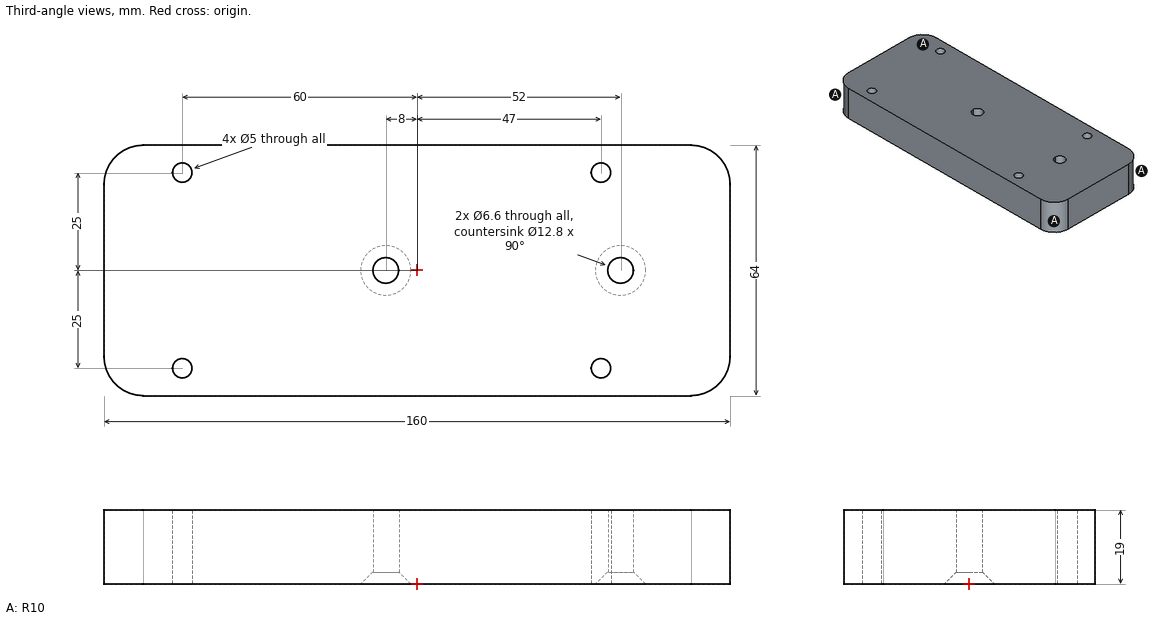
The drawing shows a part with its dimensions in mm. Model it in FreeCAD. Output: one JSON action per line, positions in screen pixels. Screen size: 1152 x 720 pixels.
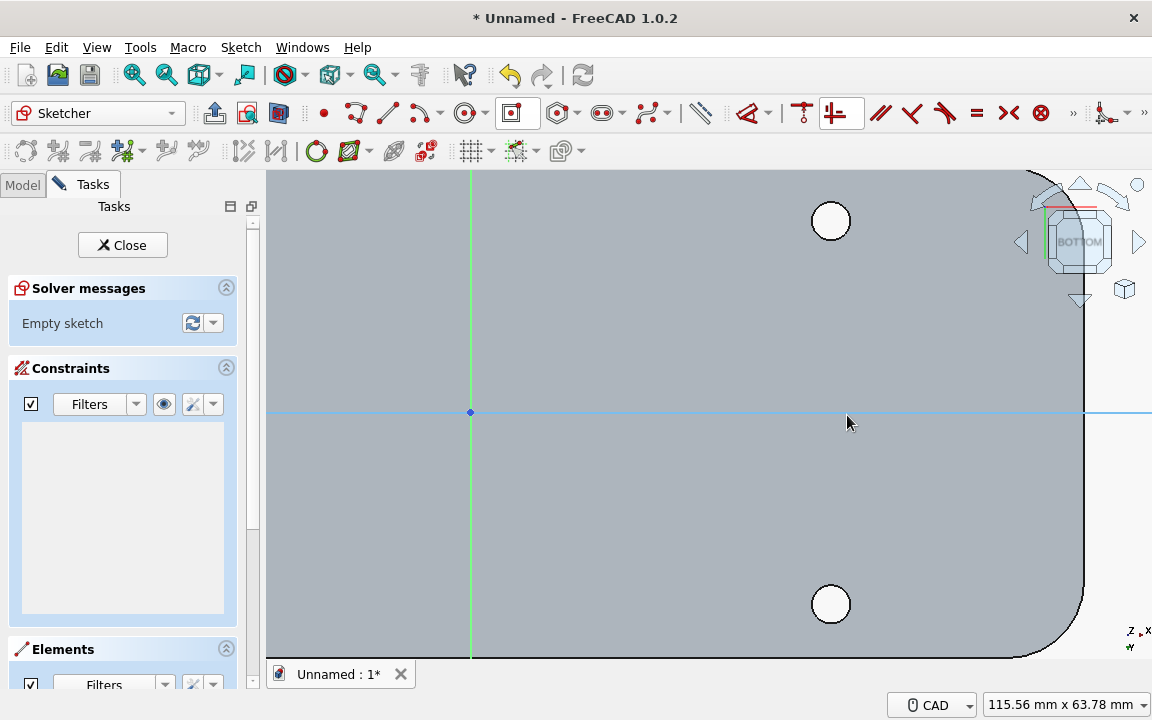
{"action": "left_click", "coordinate": [466, 114]}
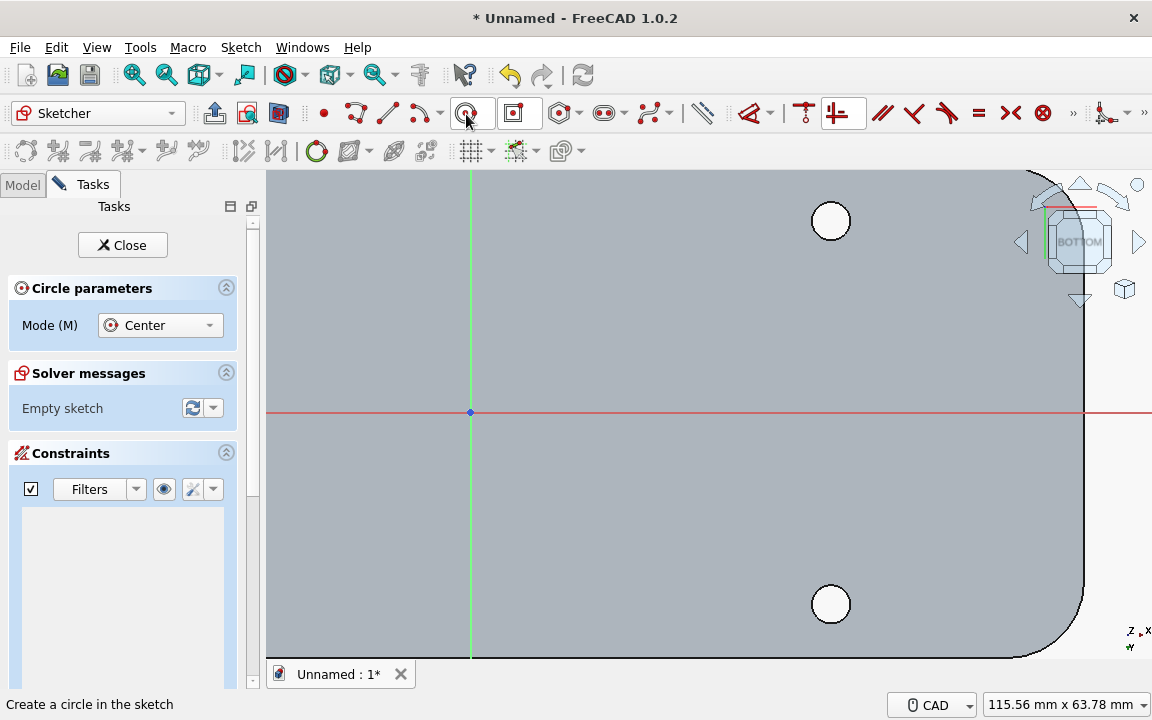
{"action": "left_click", "coordinate": [869, 413]}
{"action": "left_click", "coordinate": [887, 395]}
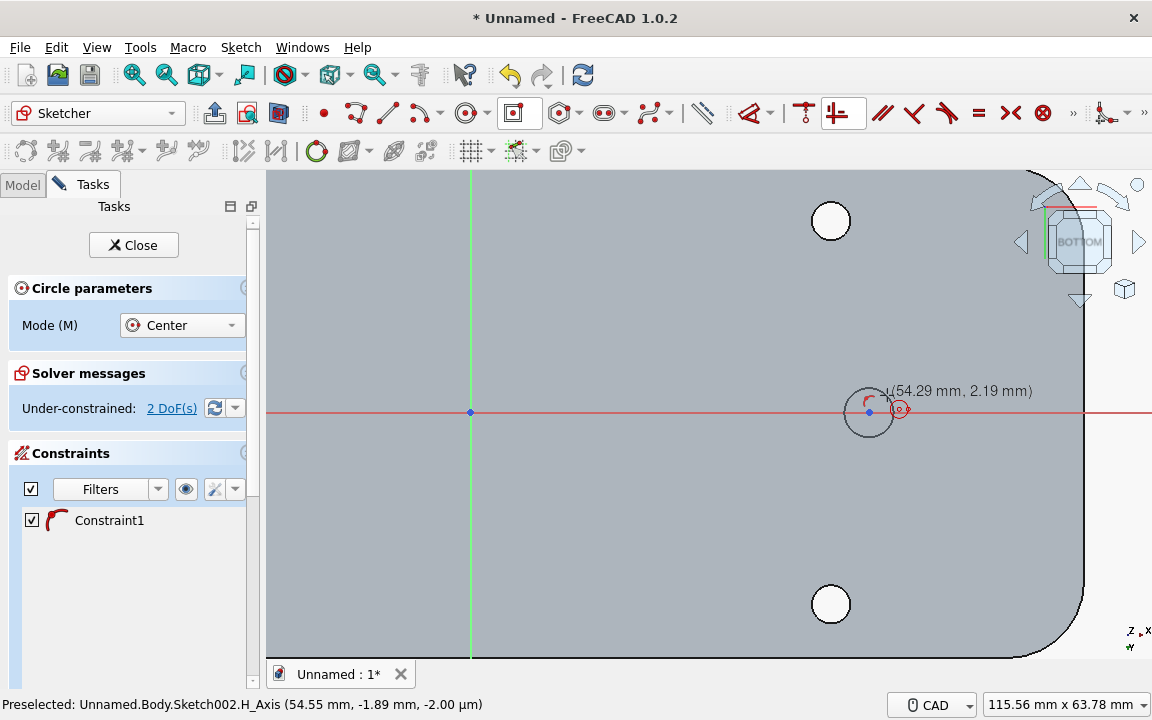
{"action": "left_click", "coordinate": [409, 413]}
{"action": "left_click", "coordinate": [427, 395]}
{"action": "key", "text": "Escape"}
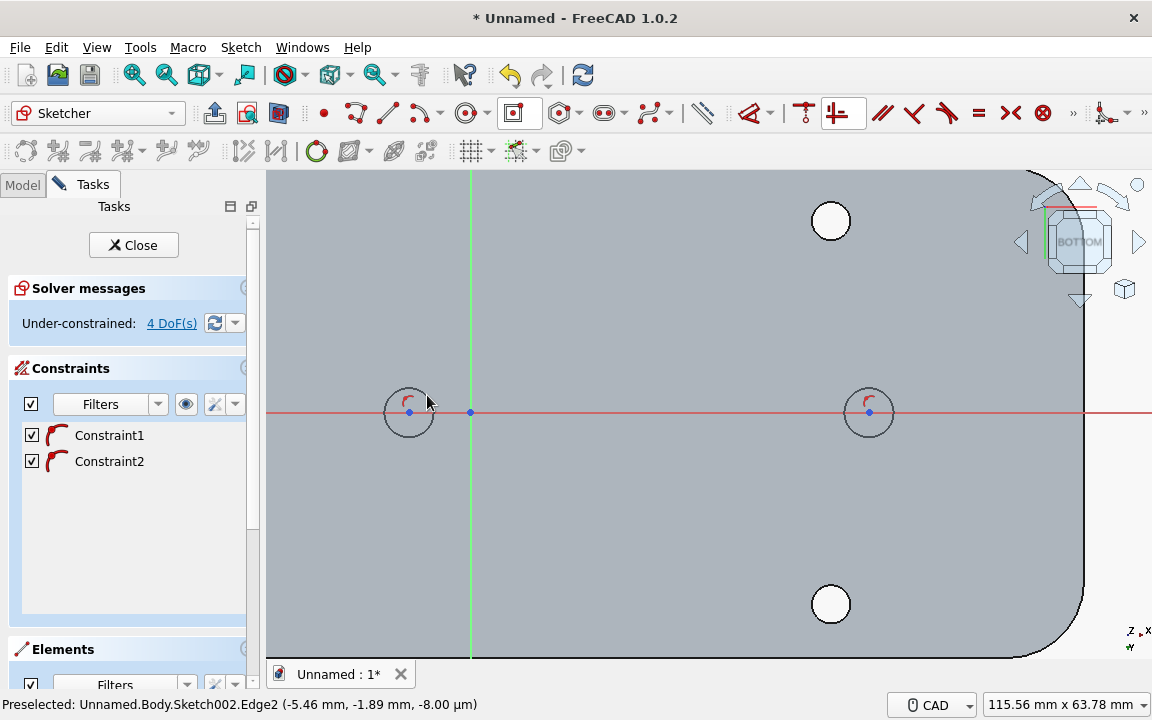
{"action": "left_click", "coordinate": [886, 395]}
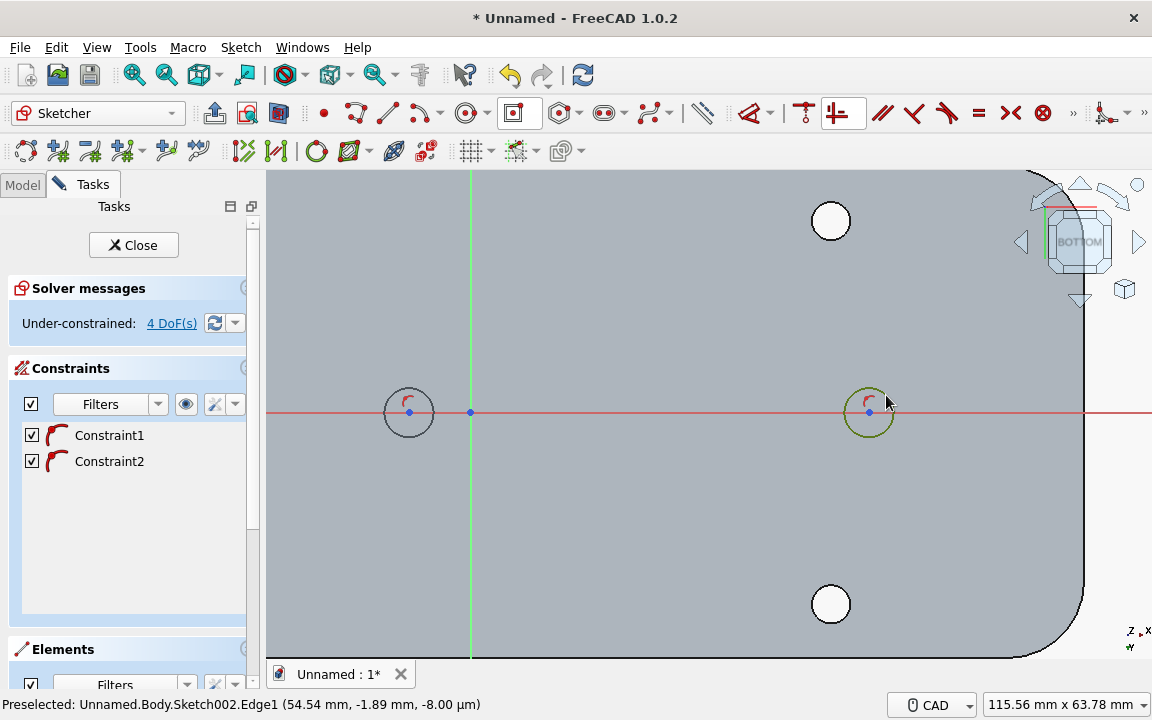
{"action": "left_click", "coordinate": [426, 395]}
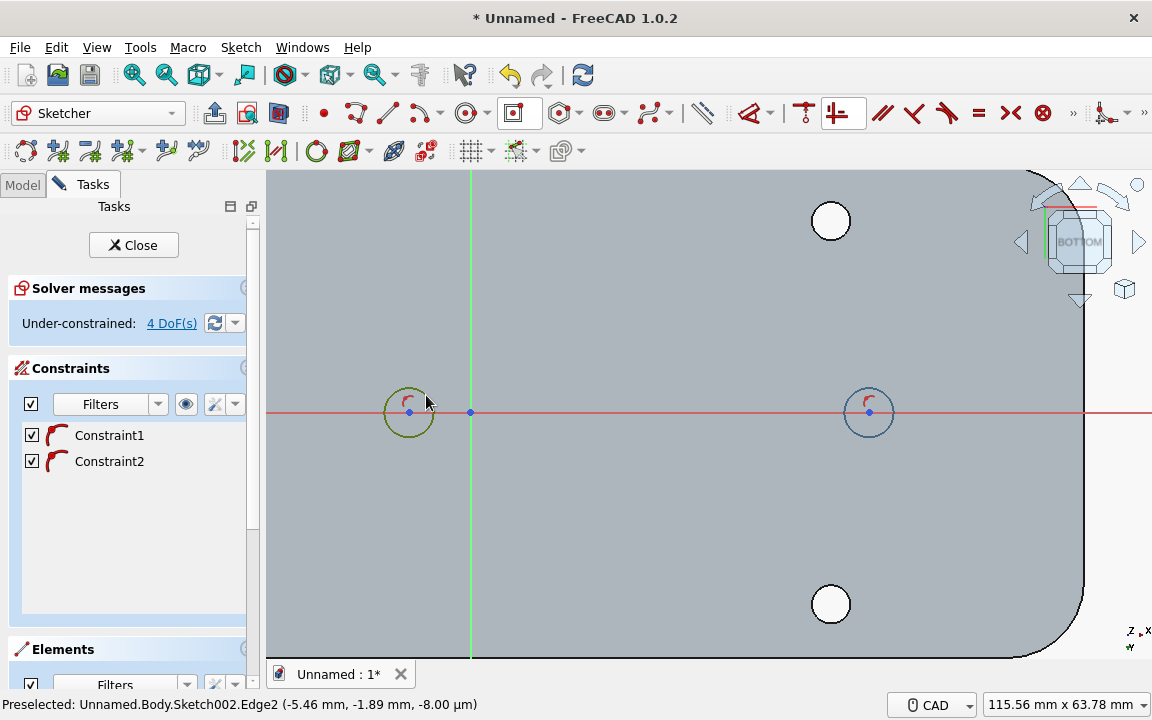
{"action": "left_click", "coordinate": [980, 114]}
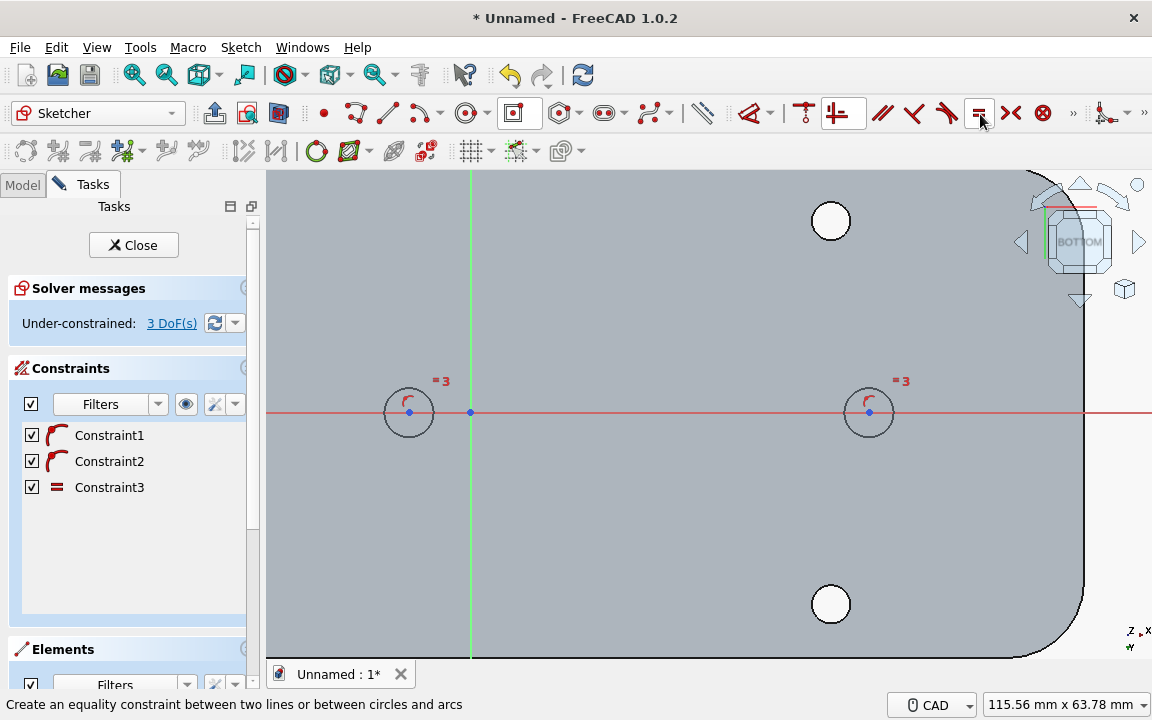
{"action": "left_click", "coordinate": [750, 114]}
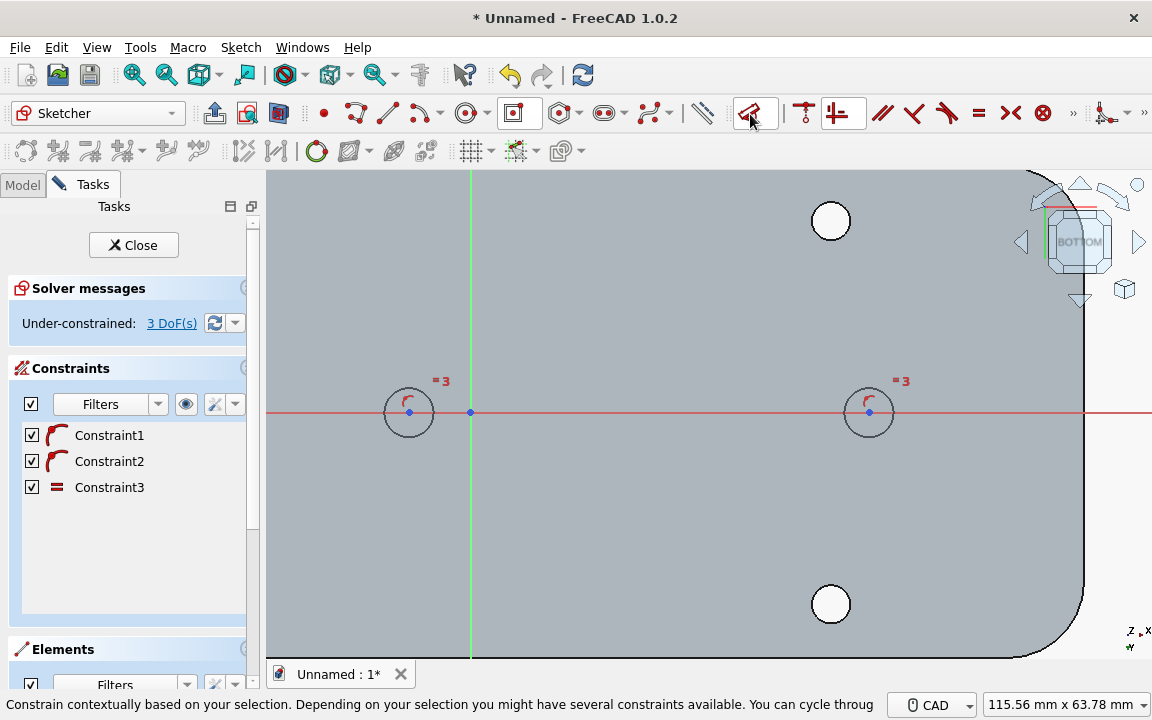
{"action": "left_click", "coordinate": [886, 395]}
{"action": "left_click", "coordinate": [908, 372]}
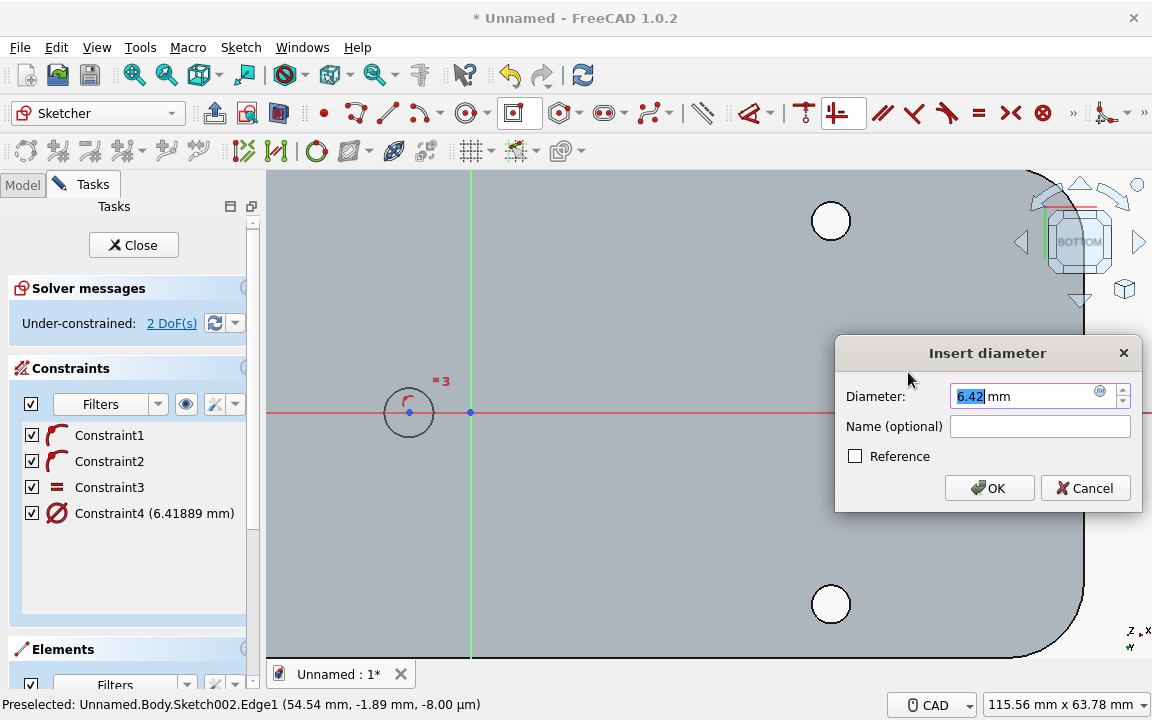
{"action": "type", "text": "6.6"}
{"action": "key", "text": "Return"}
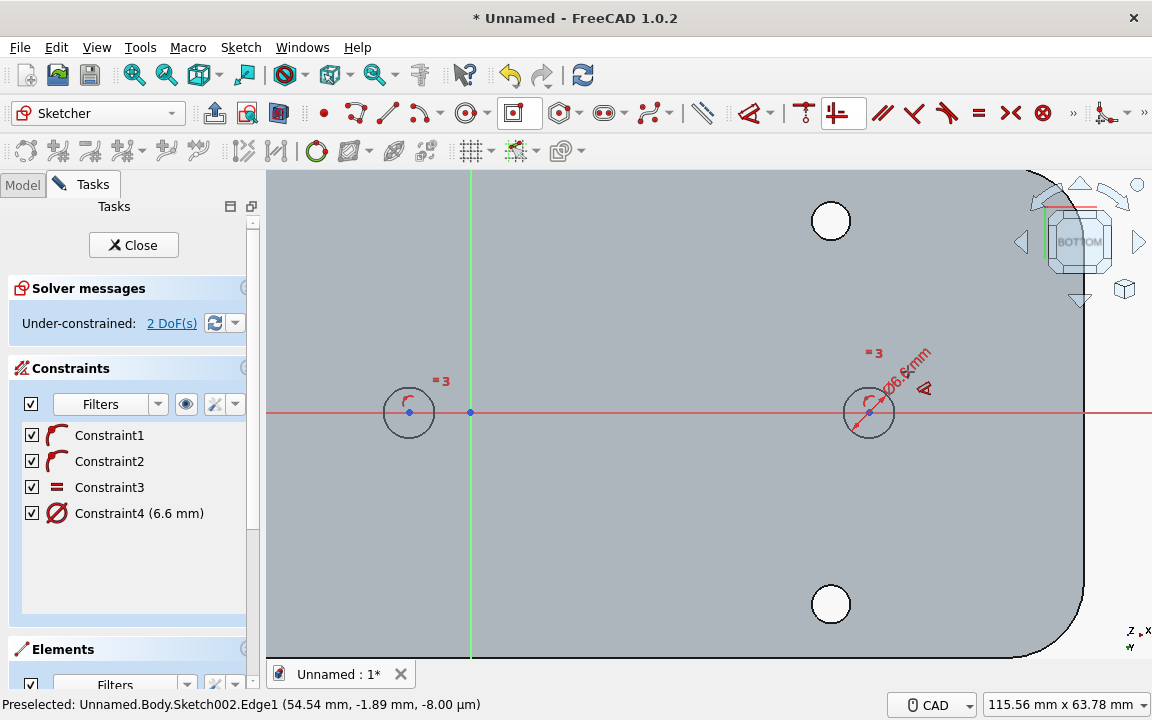
{"action": "left_click", "coordinate": [409, 413]}
{"action": "left_click", "coordinate": [440, 447]}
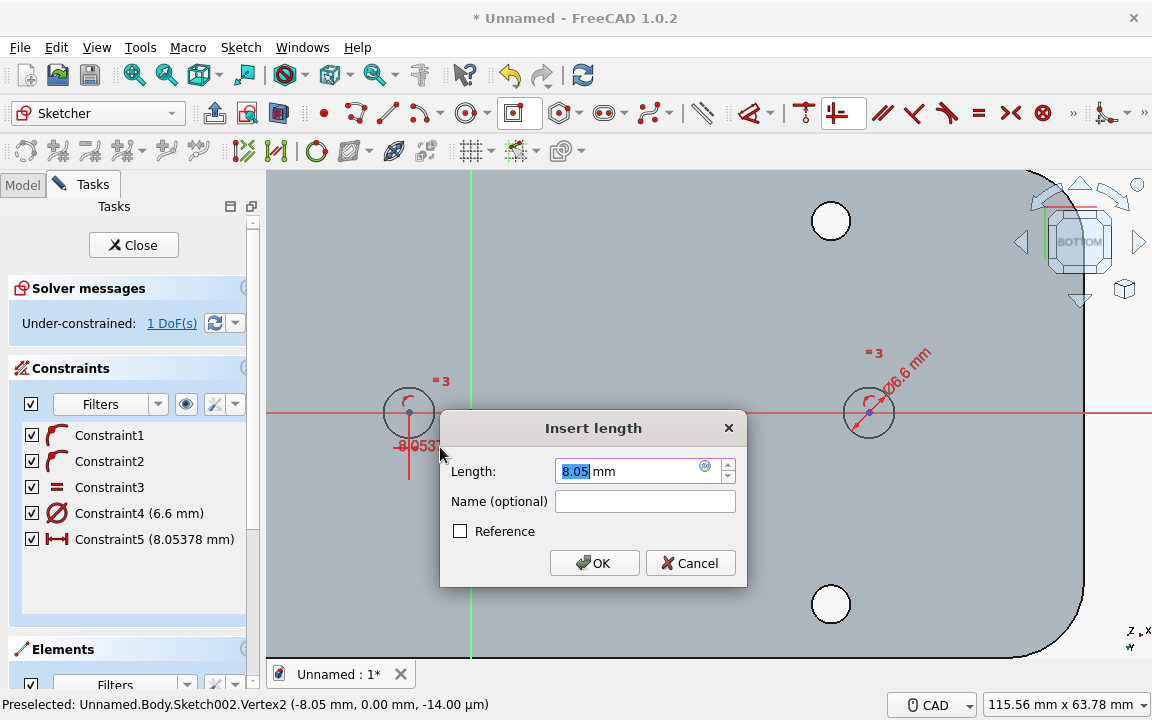
{"action": "type", "text": "8"}
{"action": "key", "text": "Return"}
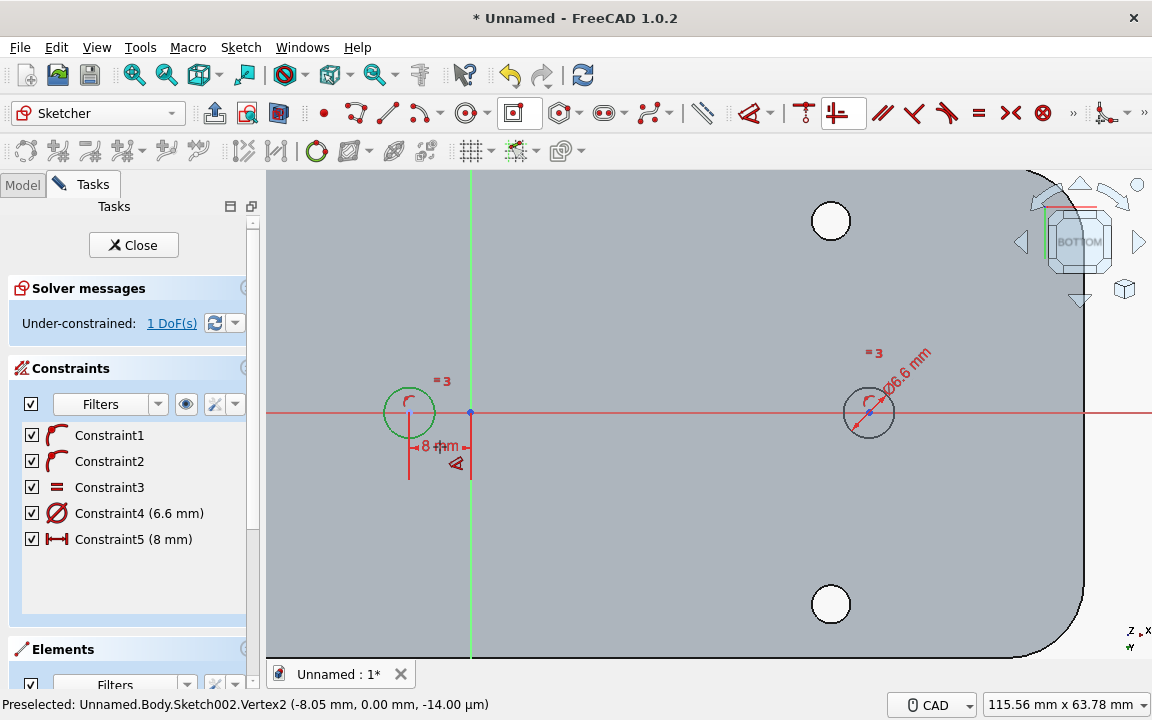
{"action": "left_click", "coordinate": [869, 413]}
{"action": "left_click", "coordinate": [670, 447]}